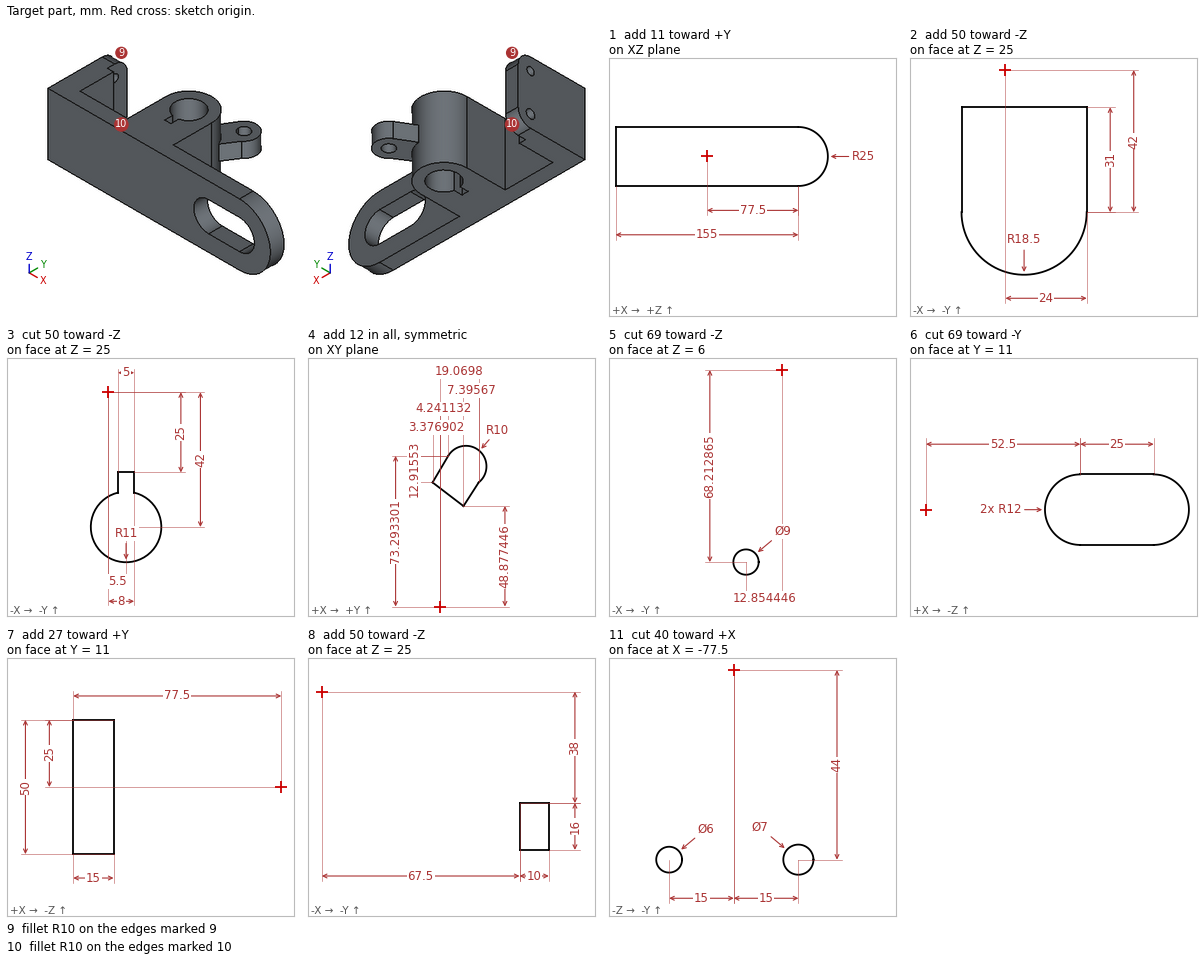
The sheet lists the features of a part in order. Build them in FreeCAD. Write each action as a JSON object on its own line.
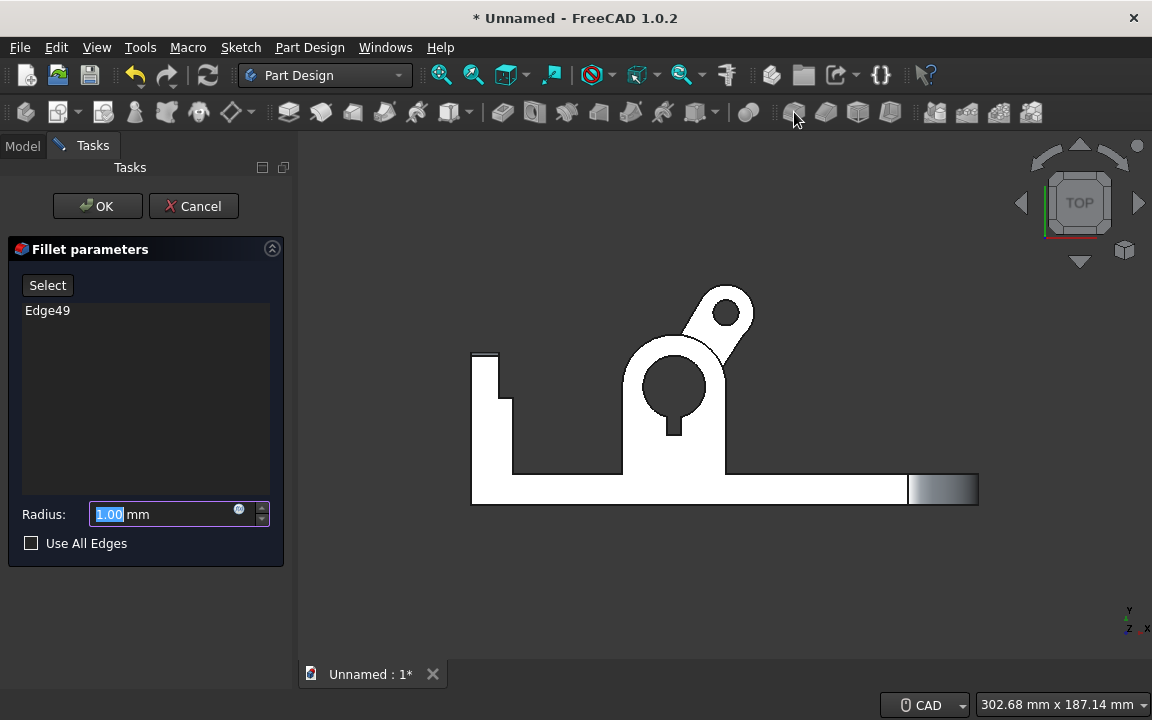
{"action": "type", "text": "10"}
{"action": "key", "text": "Tab"}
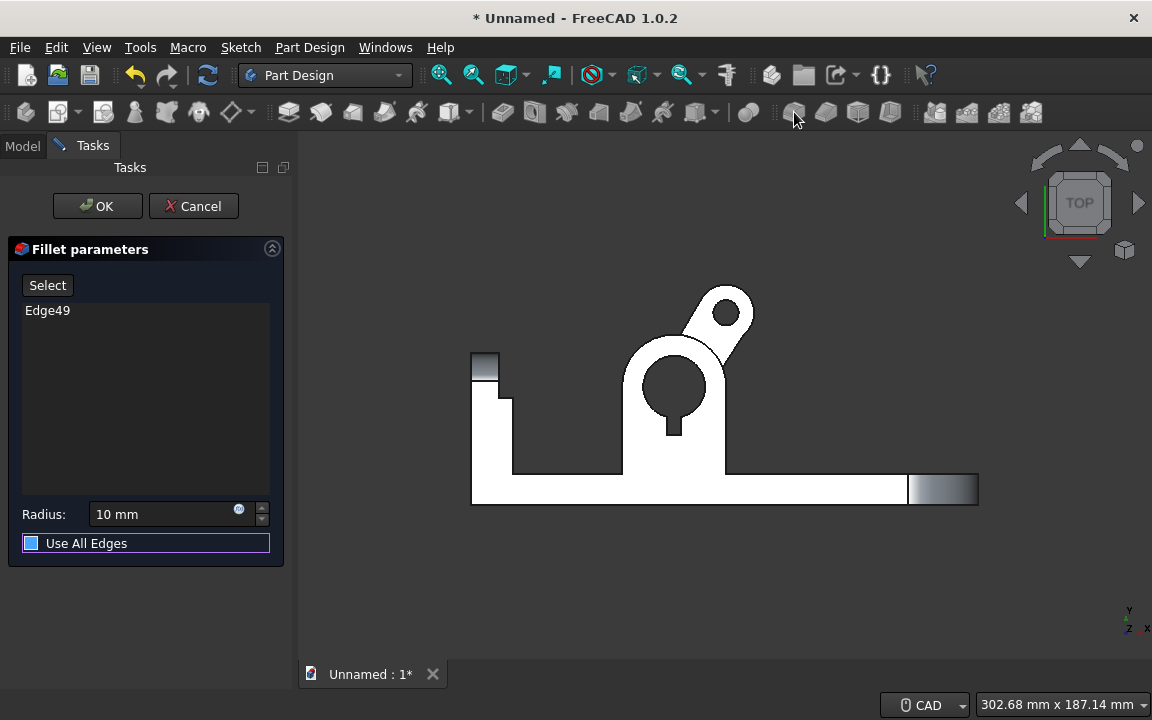
{"action": "left_click", "coordinate": [98, 206]}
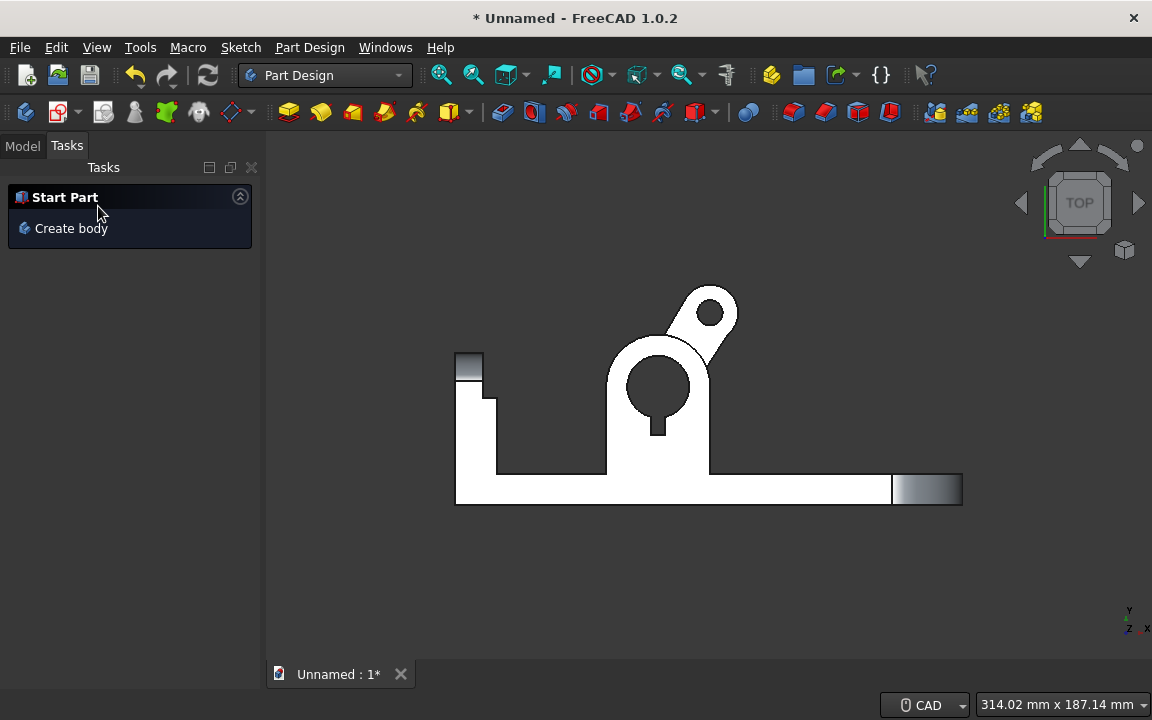
{"action": "key", "text": "0"}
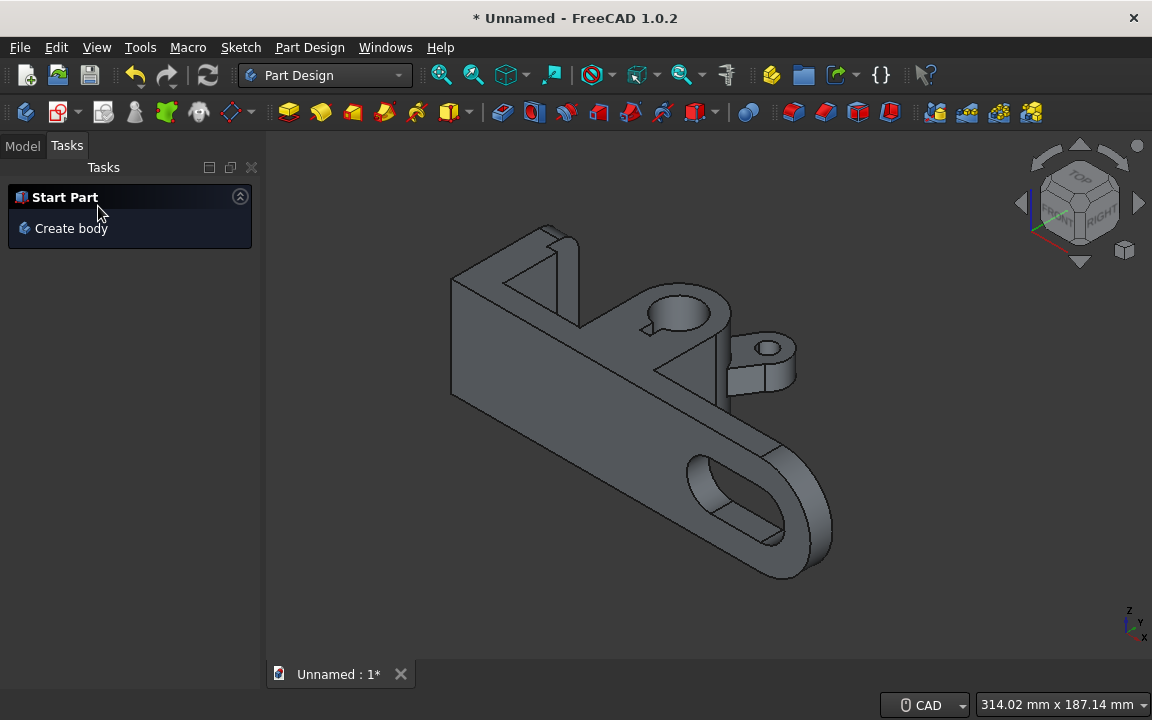
{"action": "key", "text": "2"}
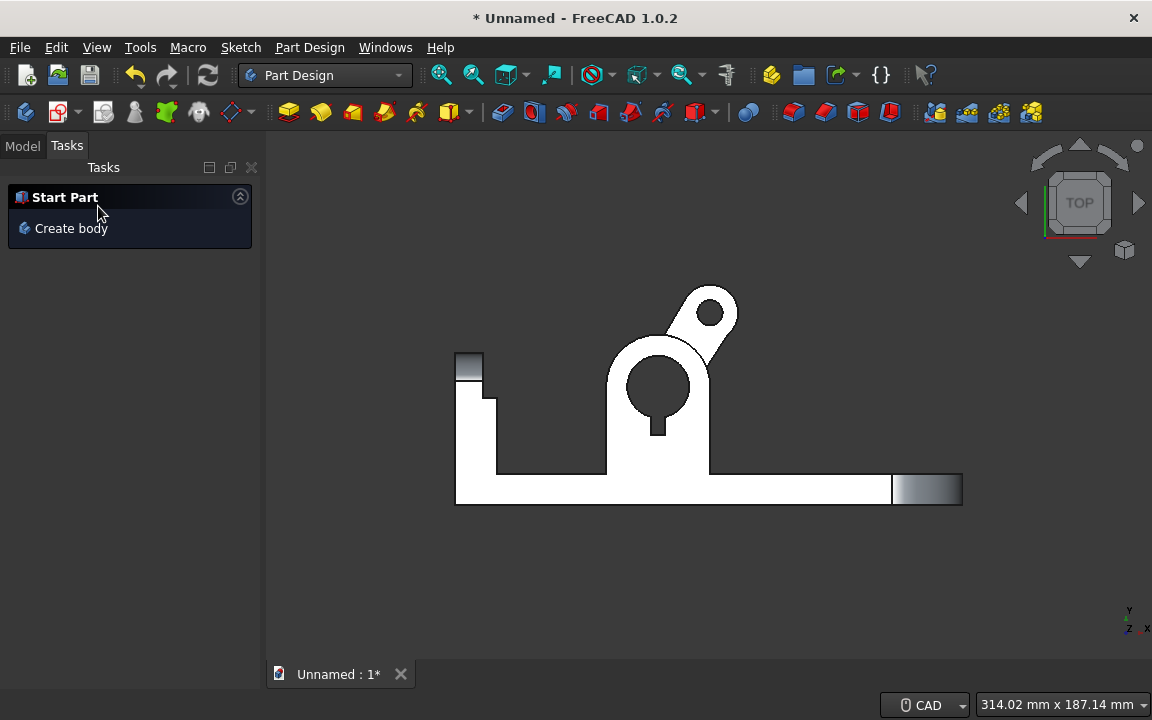
{"action": "key", "text": "1"}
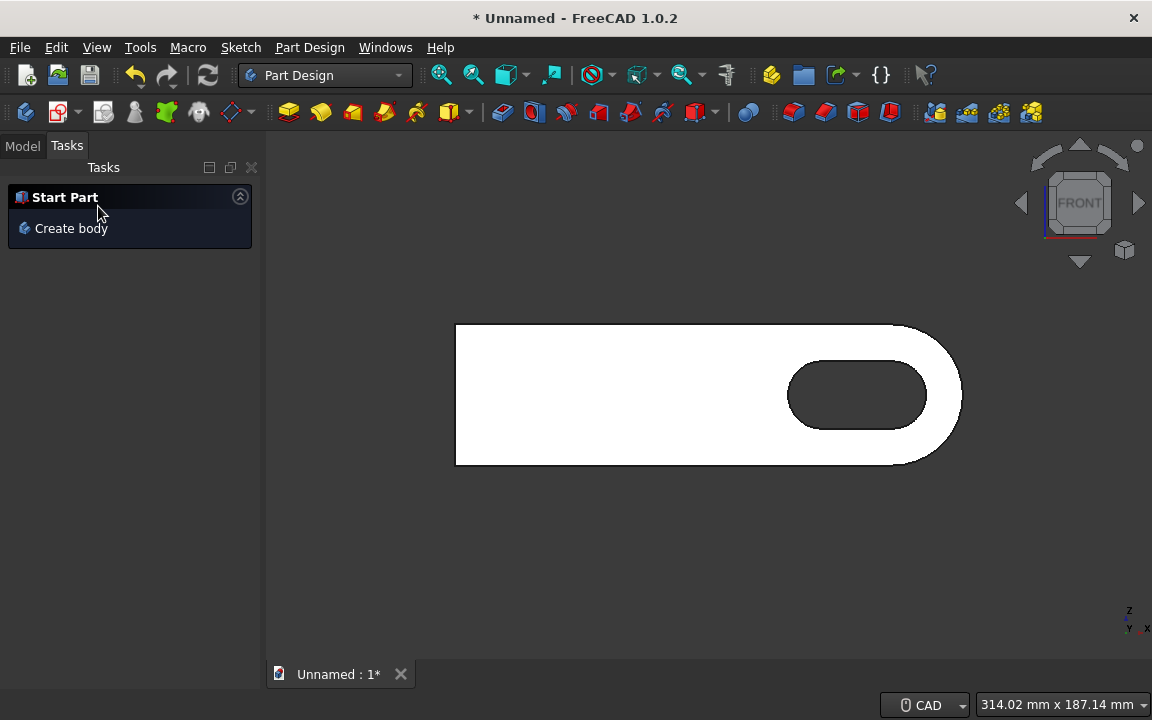
{"action": "key", "text": "3"}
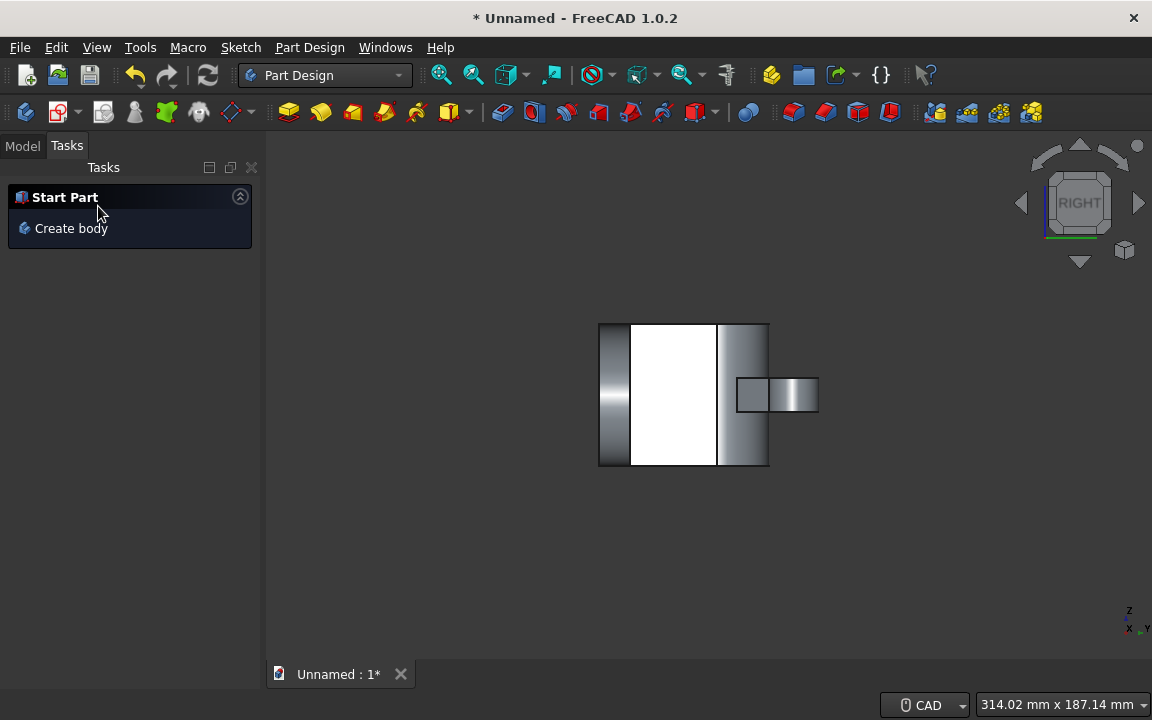
{"action": "left_click", "coordinate": [442, 76]}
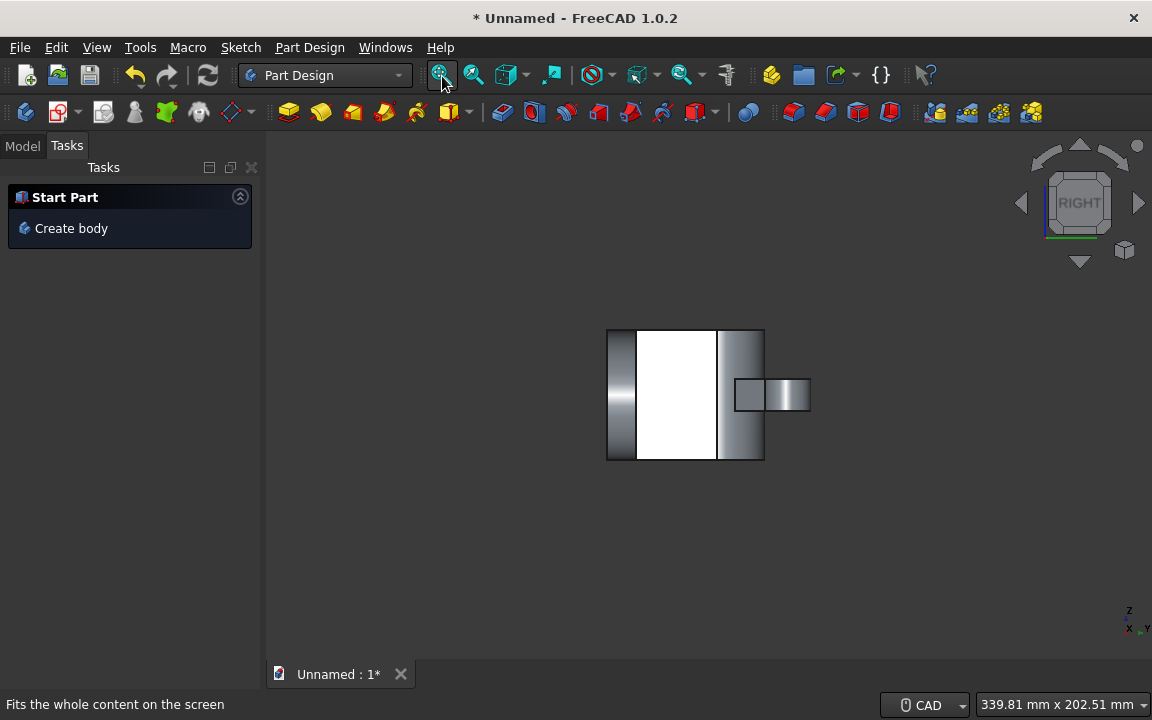
{"action": "key", "text": "5"}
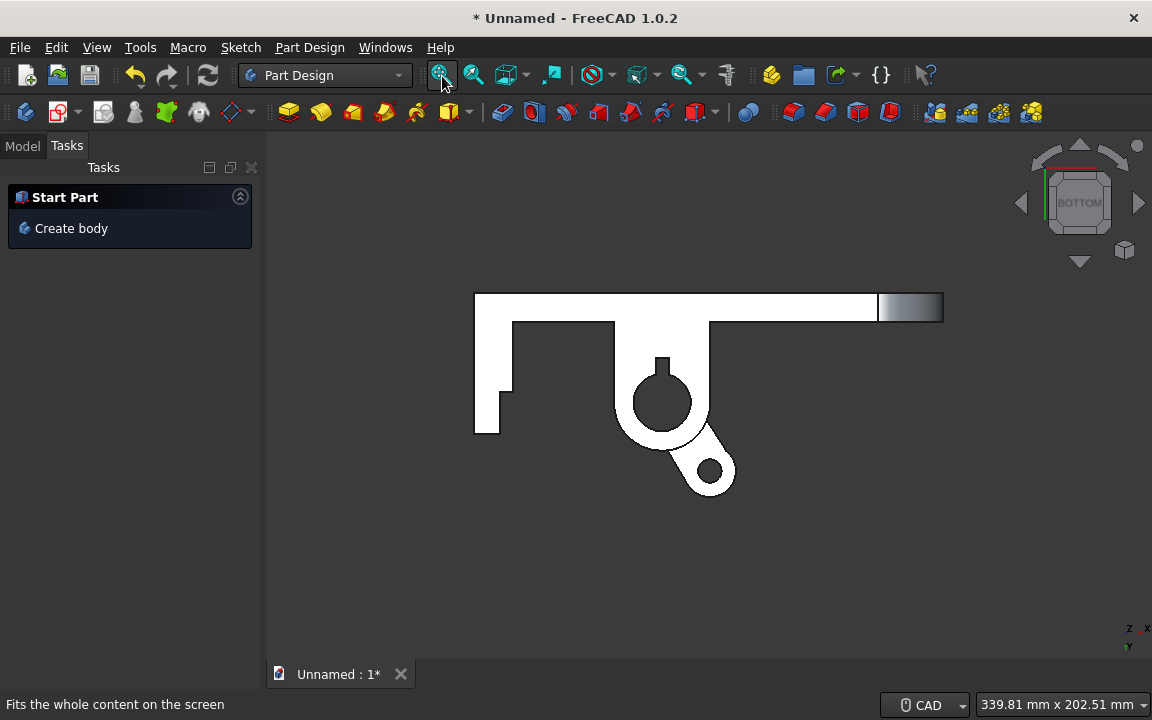
{"action": "key", "text": "4"}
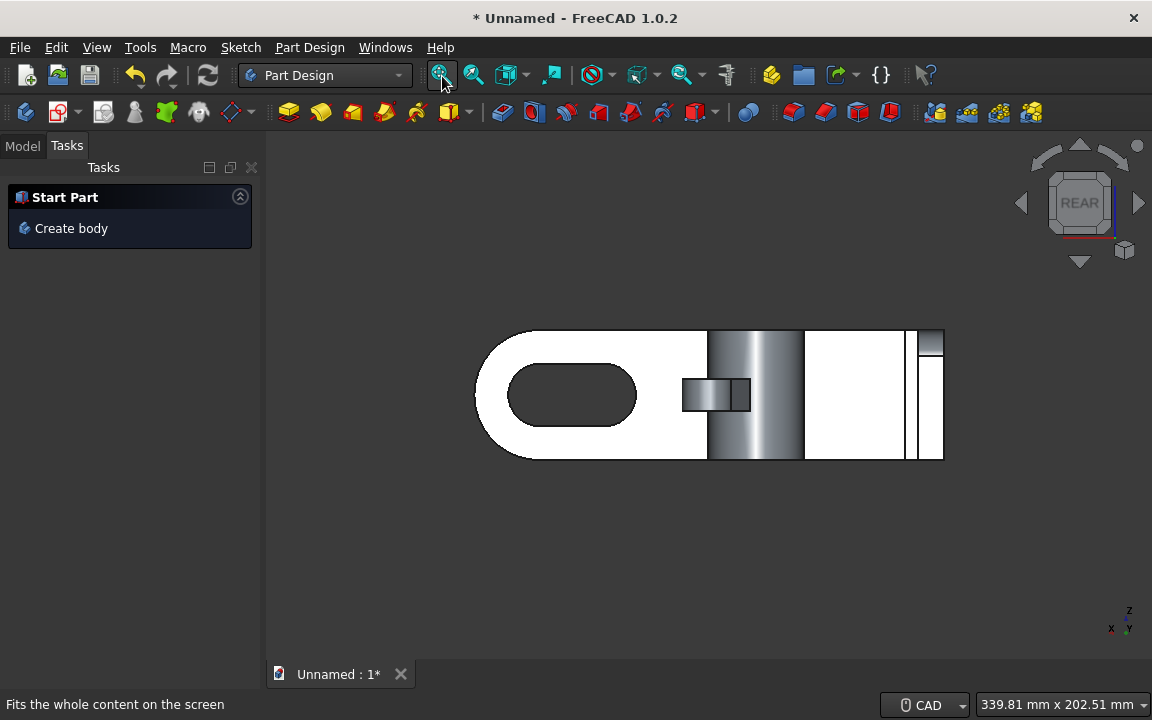
{"action": "left_click", "coordinate": [931, 459]}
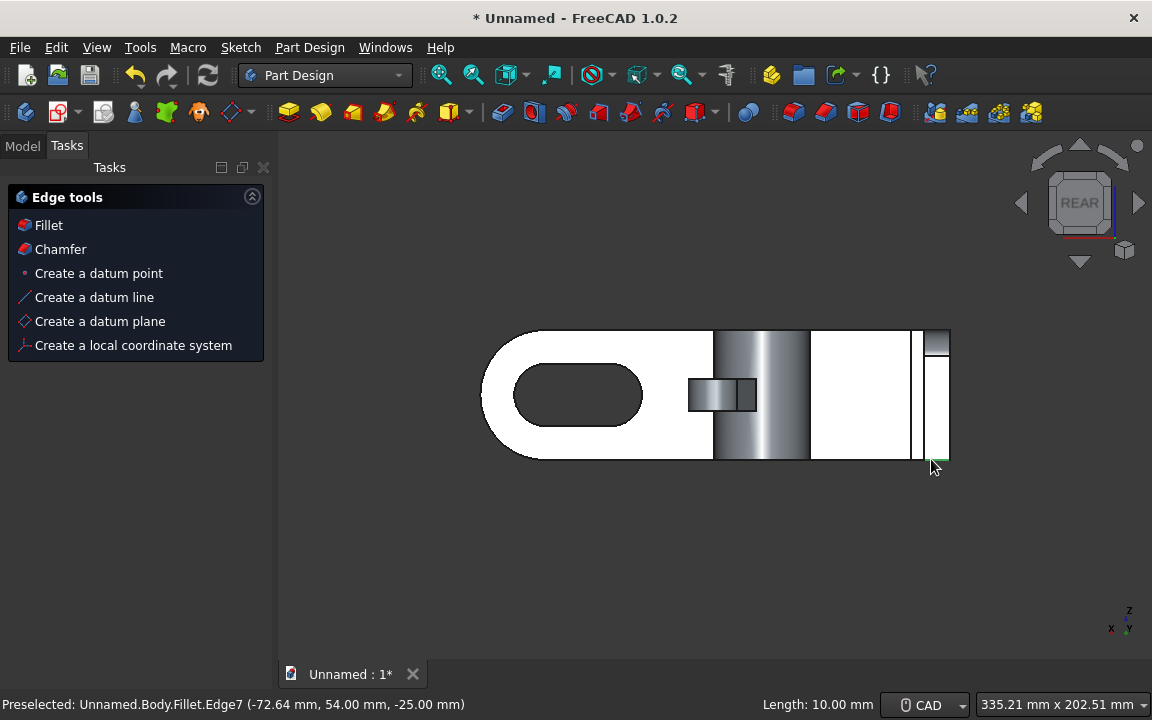
{"action": "left_click", "coordinate": [794, 112]}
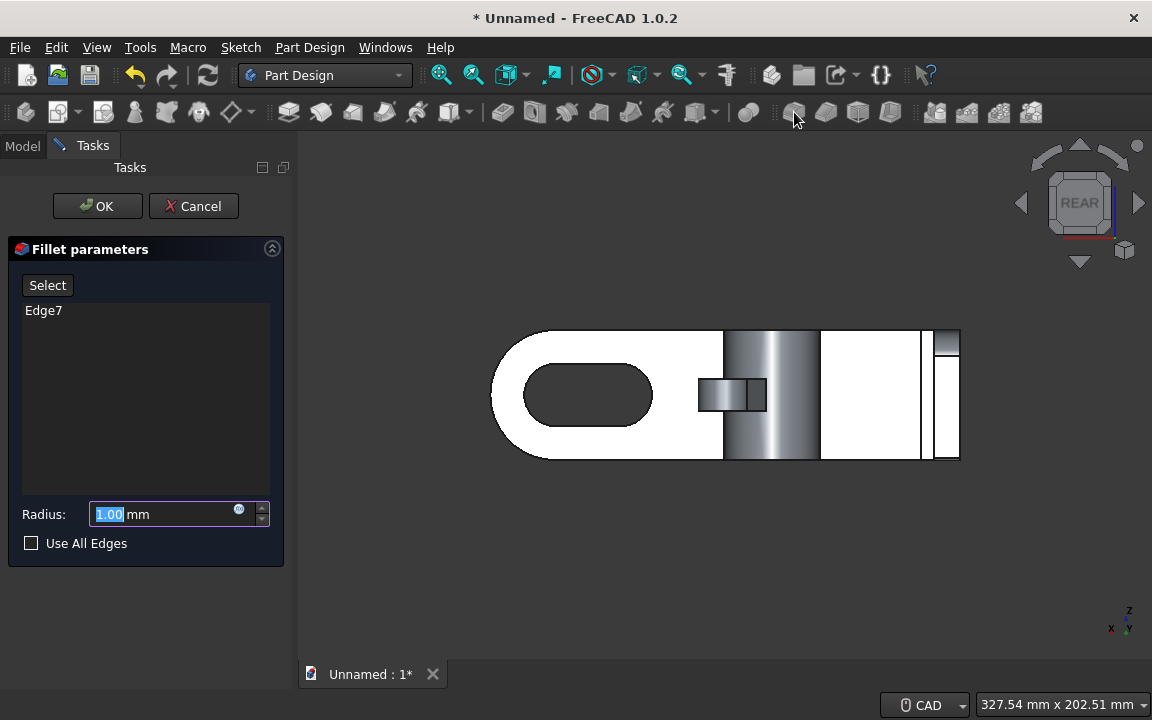
{"action": "type", "text": "10"}
{"action": "key", "text": "Tab"}